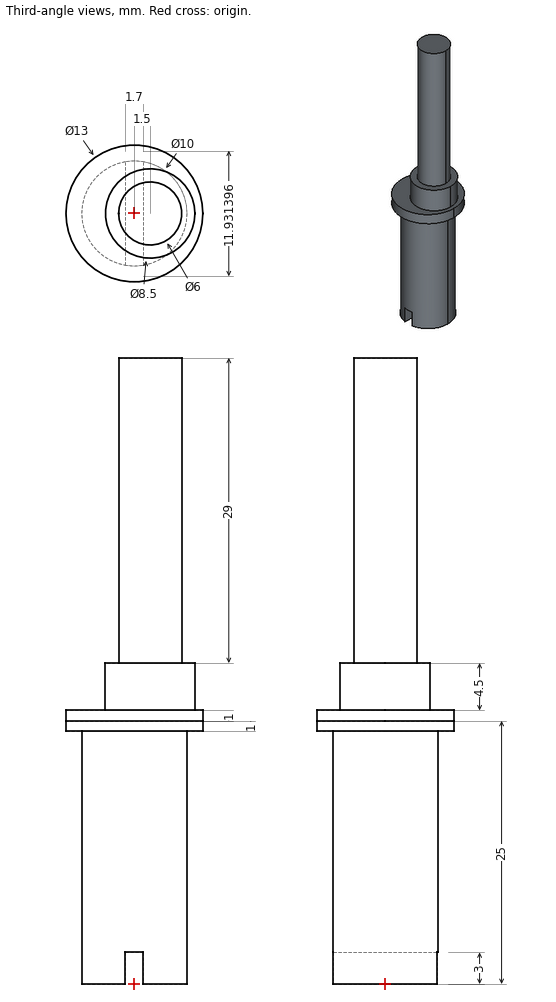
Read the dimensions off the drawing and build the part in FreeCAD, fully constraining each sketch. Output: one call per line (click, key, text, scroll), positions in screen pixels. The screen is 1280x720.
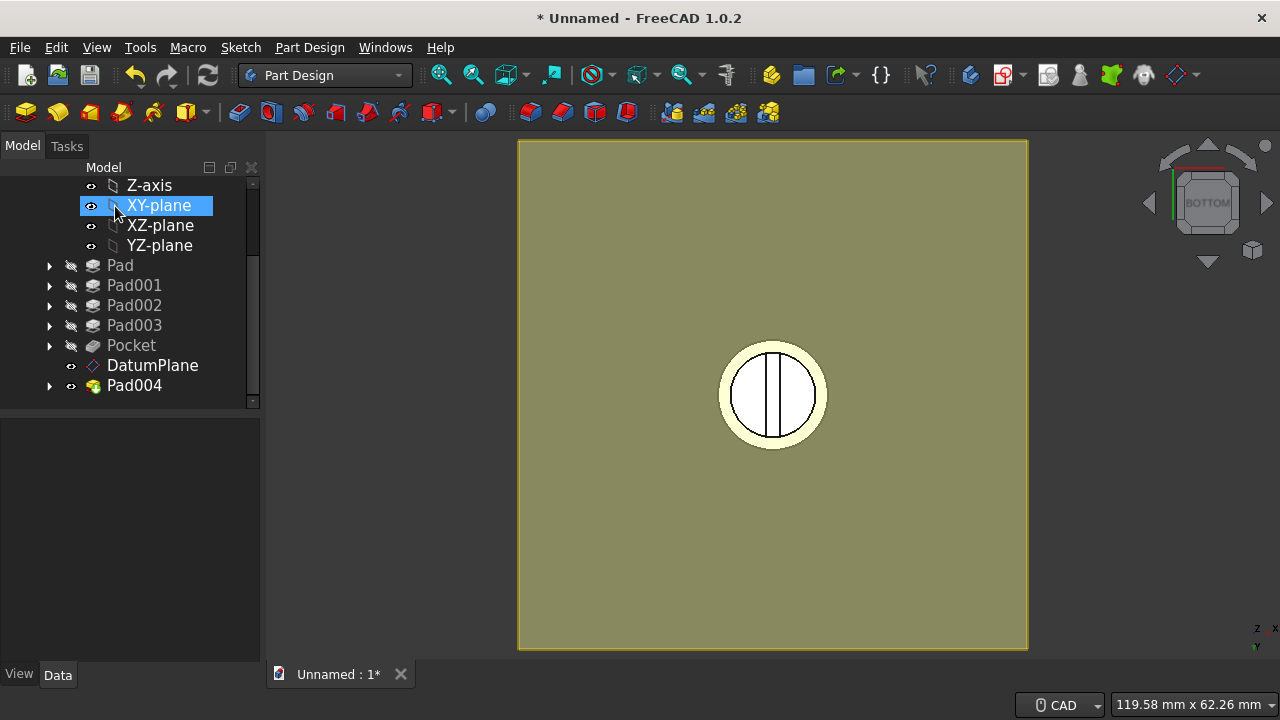
click(116, 366)
key(space)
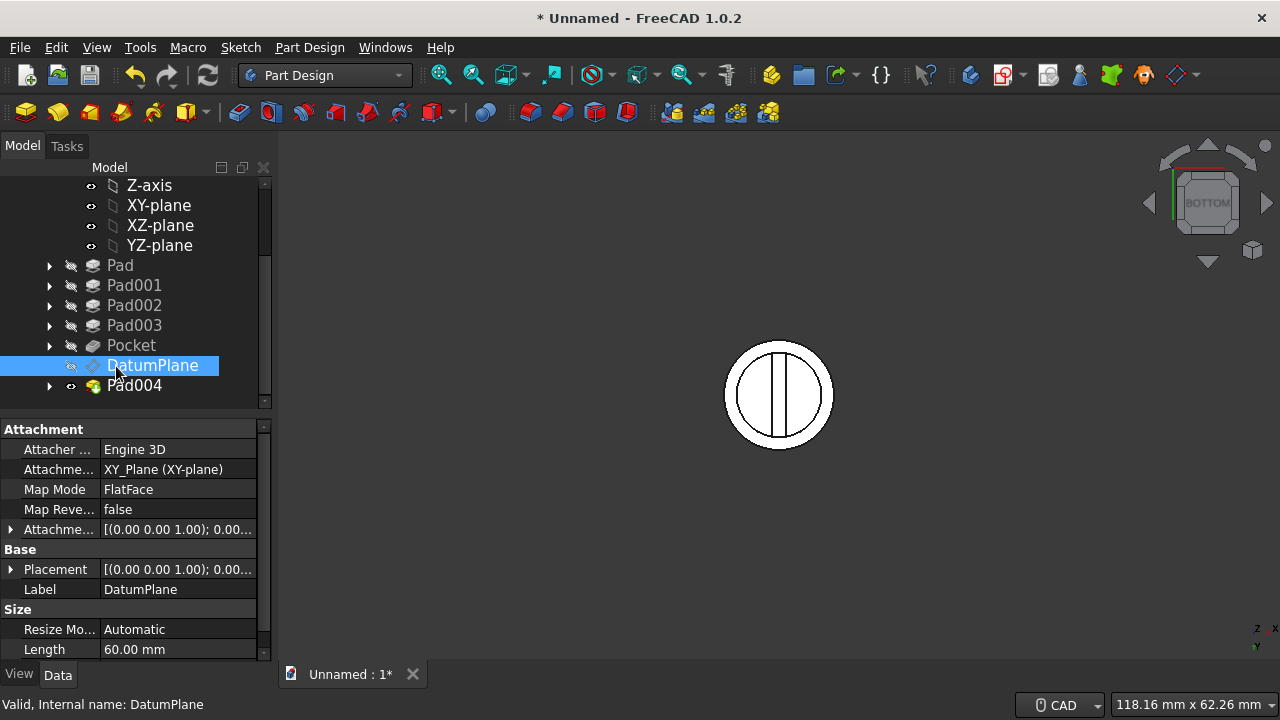
key(0)